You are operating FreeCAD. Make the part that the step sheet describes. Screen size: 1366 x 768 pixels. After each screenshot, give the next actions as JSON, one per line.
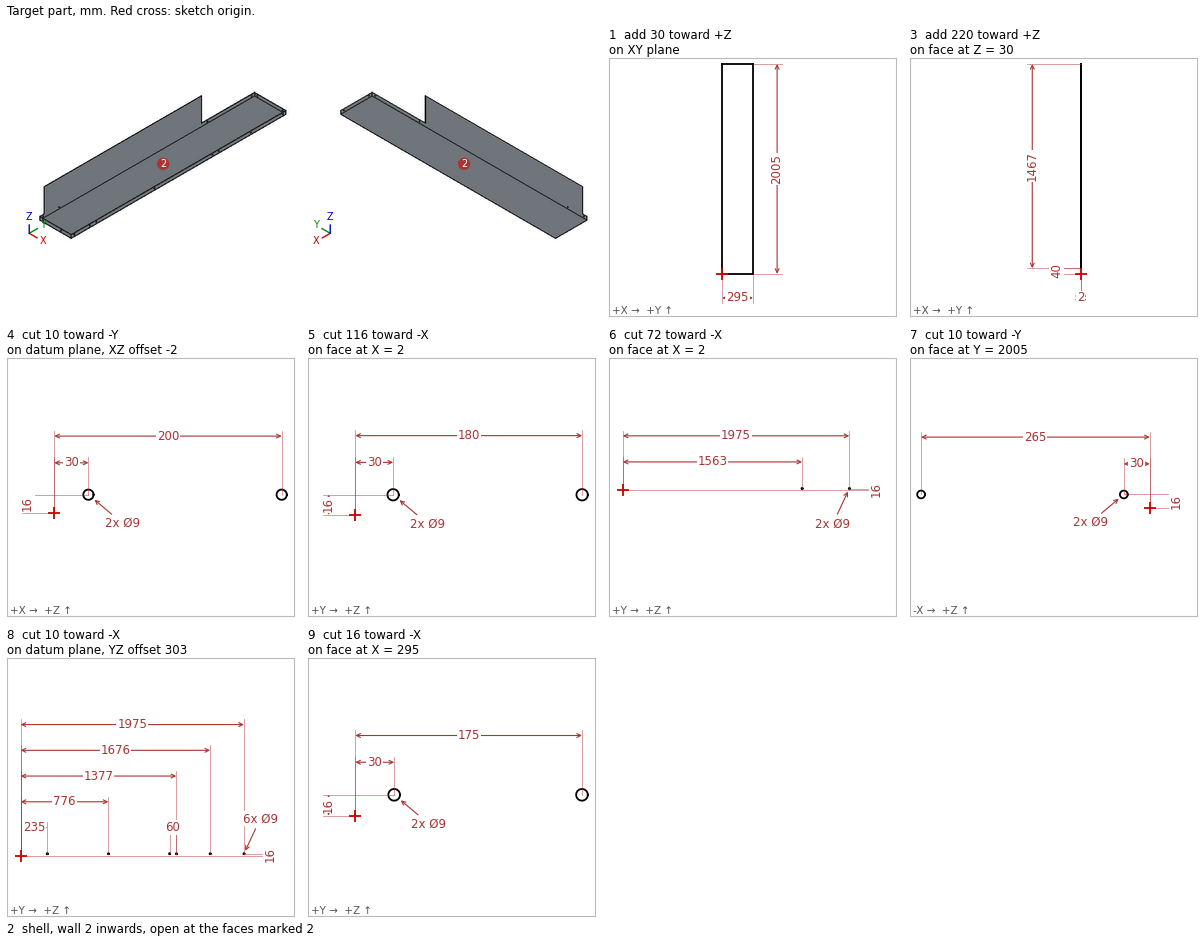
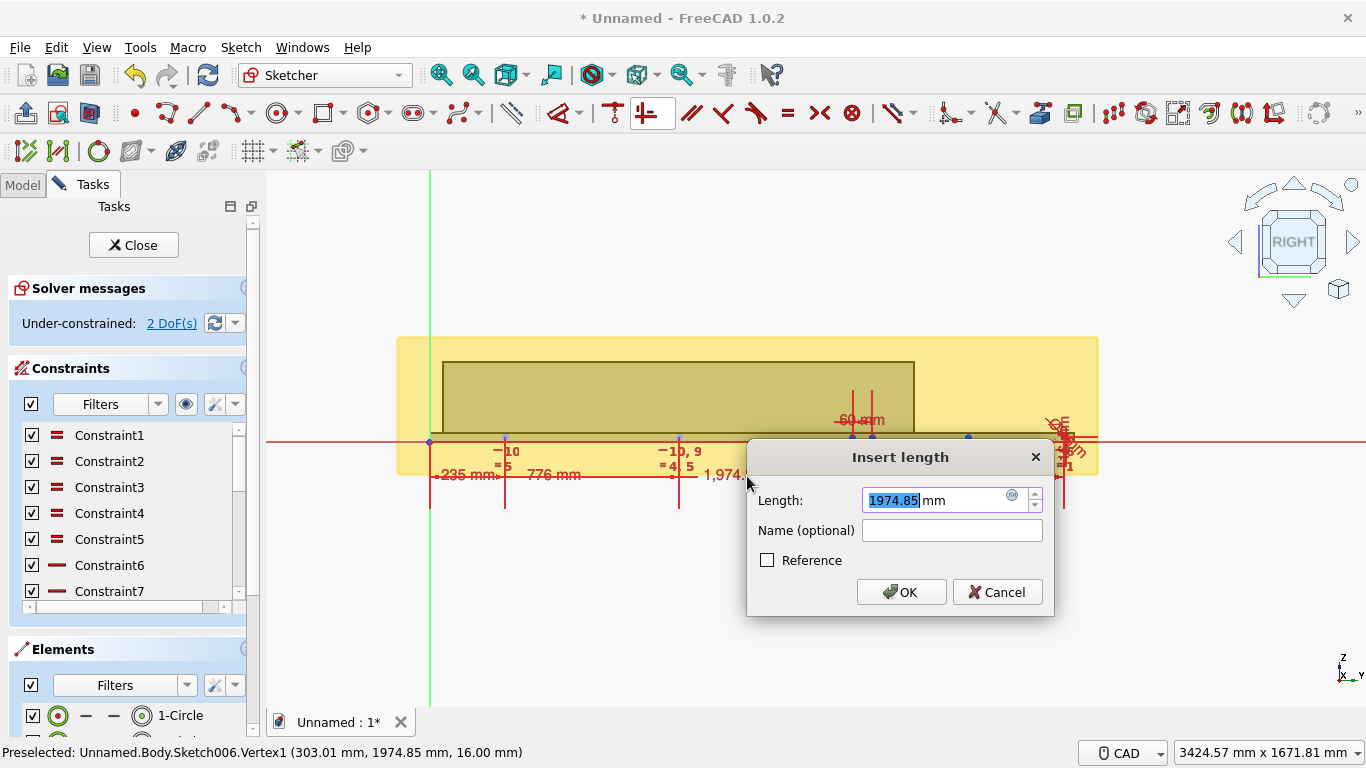
{"action": "type", "text": "1975"}
{"action": "key", "text": "Return"}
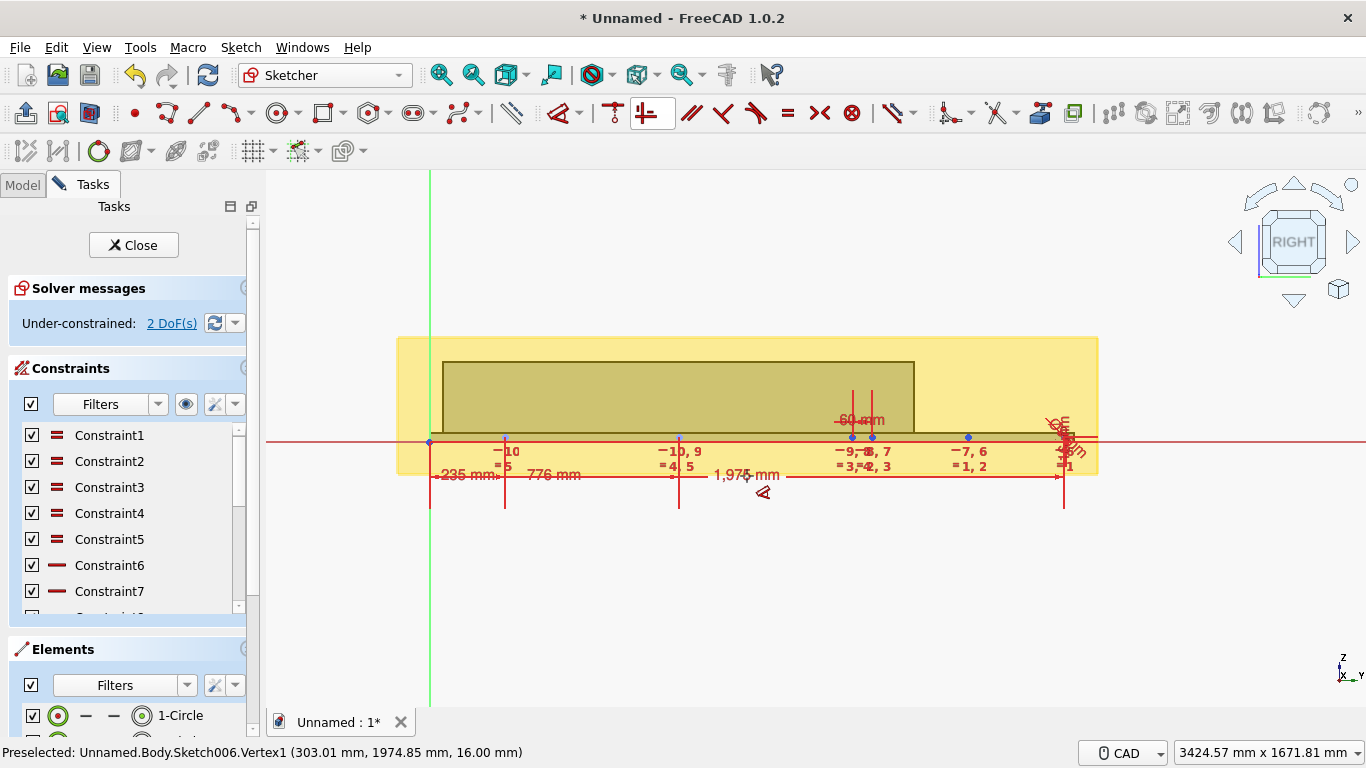
{"action": "left_click", "coordinate": [968, 437]}
{"action": "left_click", "coordinate": [823, 476]}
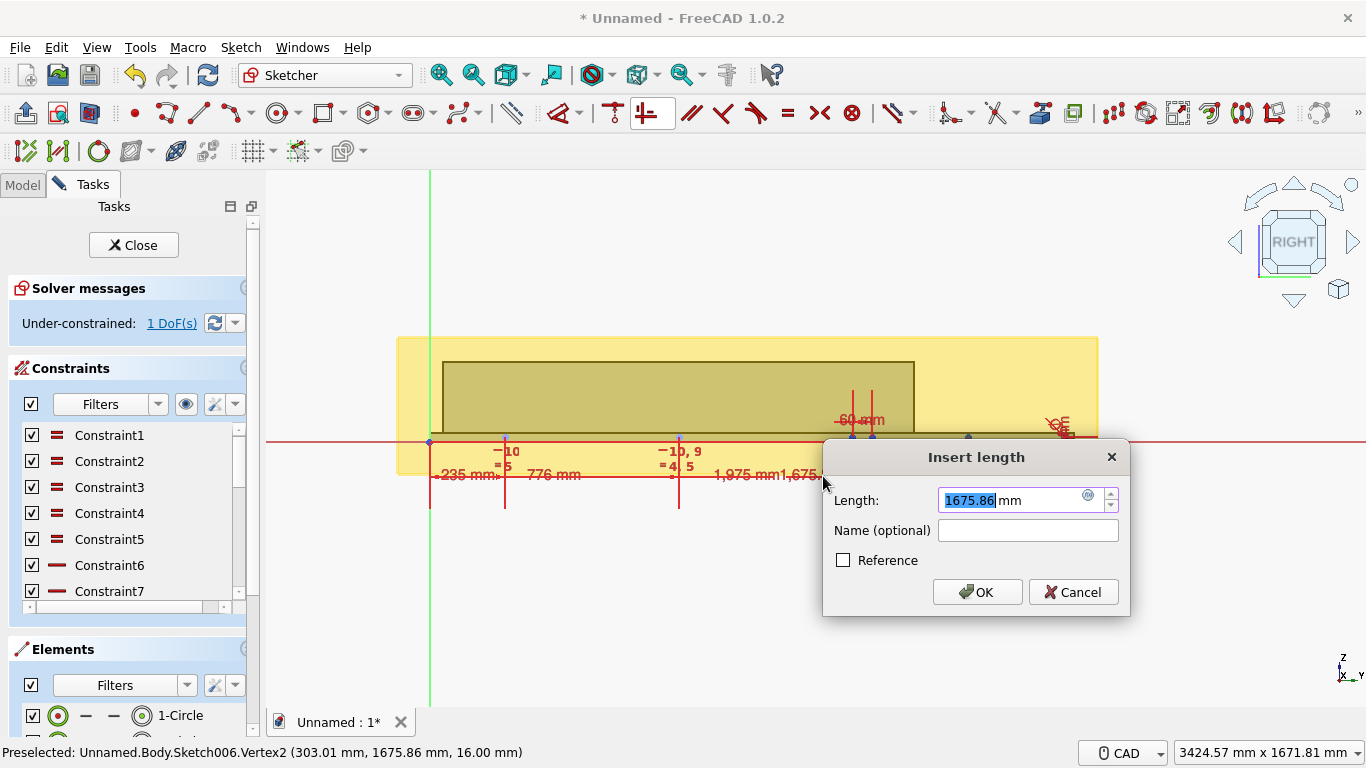
{"action": "type", "text": "1676"}
{"action": "key", "text": "Return"}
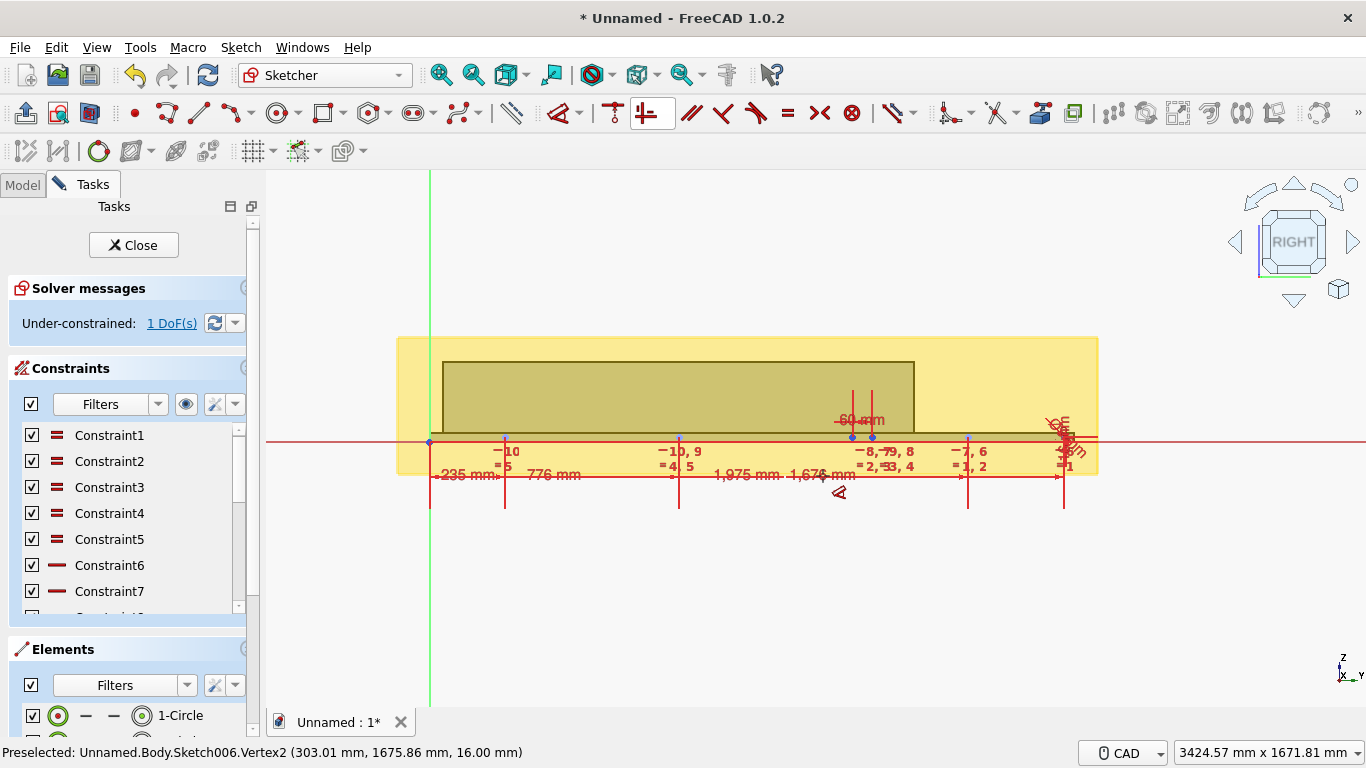
{"action": "left_click", "coordinate": [872, 437]}
{"action": "left_click", "coordinate": [651, 476]}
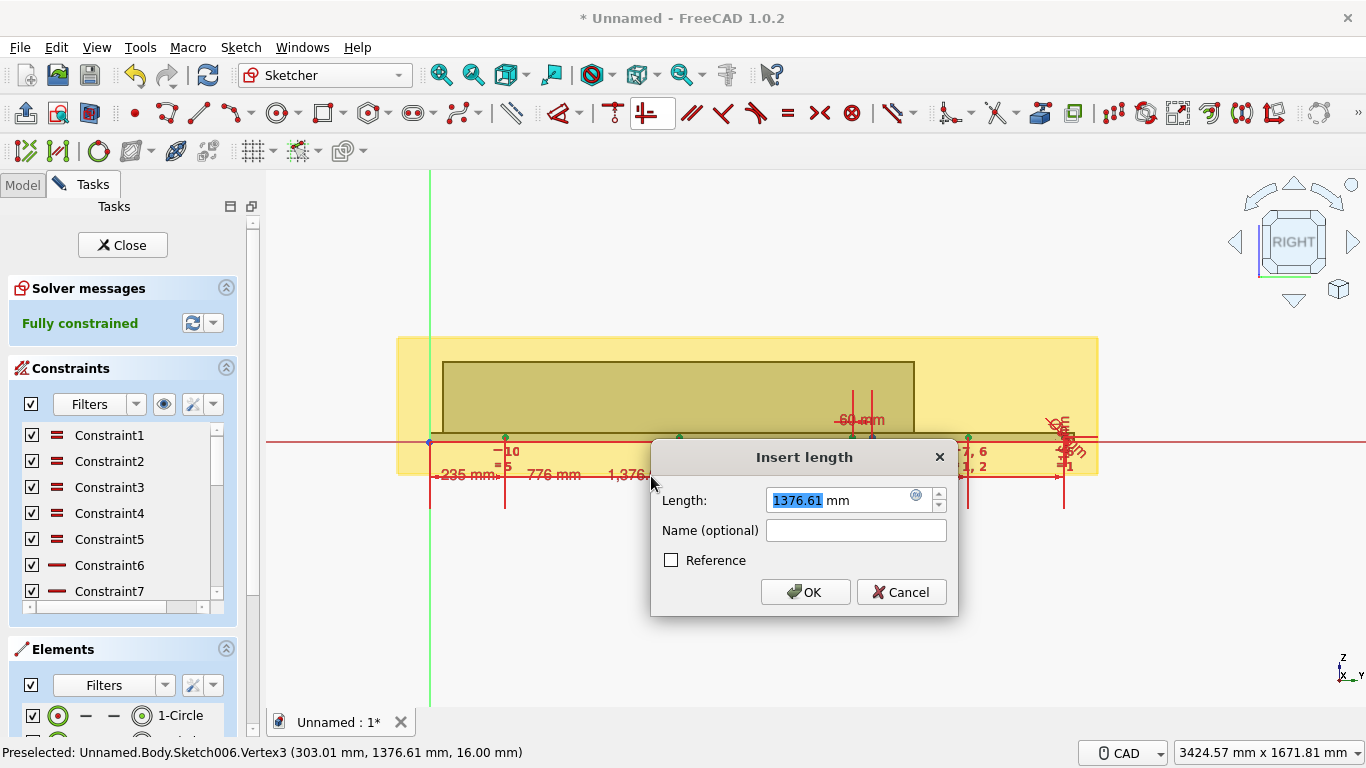
{"action": "type", "text": "1377"}
{"action": "key", "text": "Return"}
{"action": "key", "text": "Escape"}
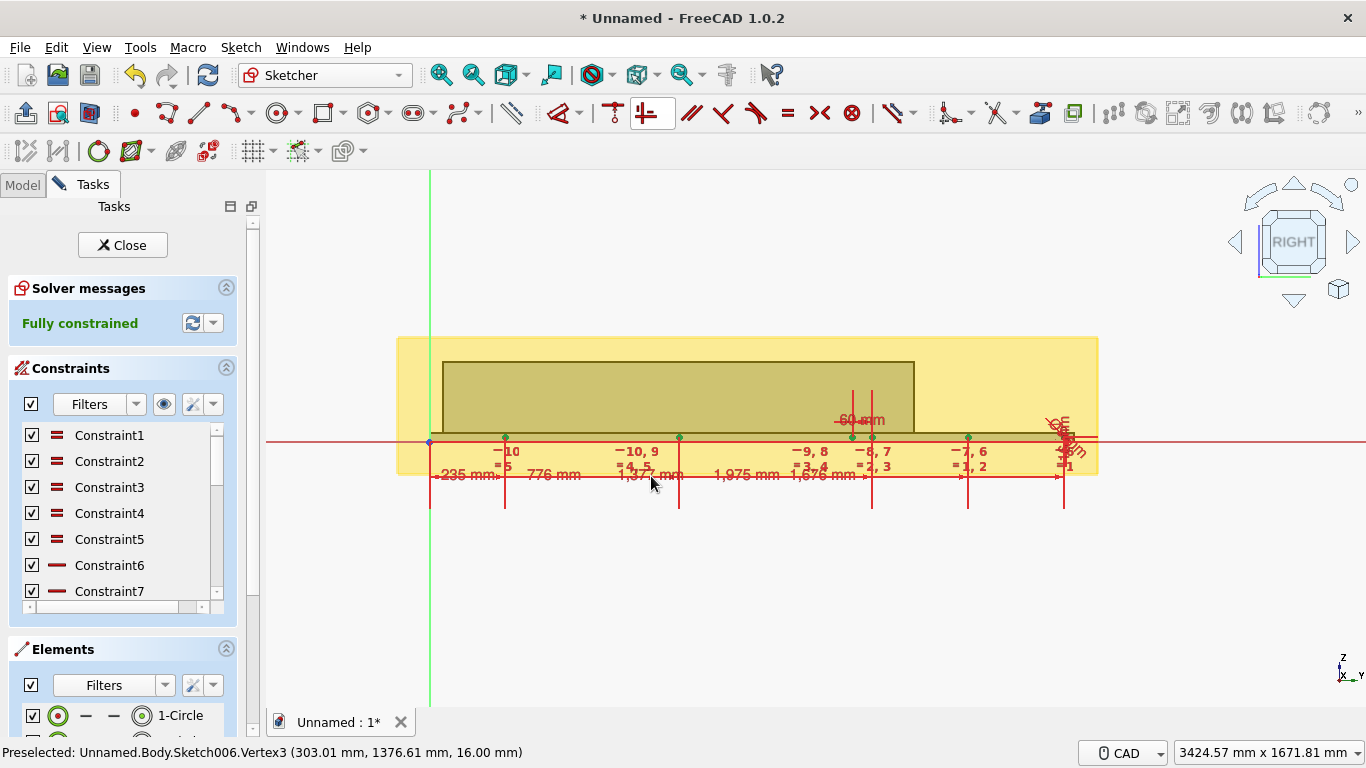
{"action": "left_click", "coordinate": [123, 245]}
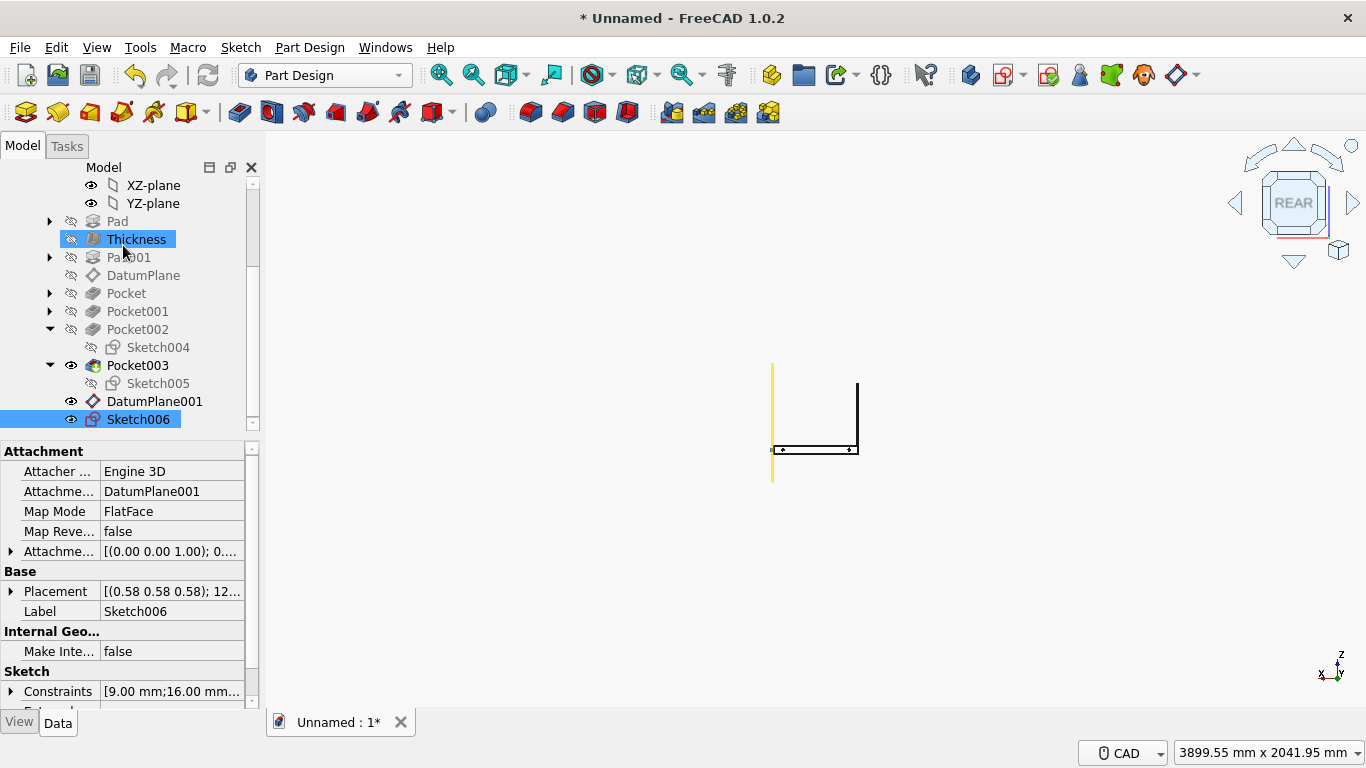
{"action": "left_click", "coordinate": [240, 112]}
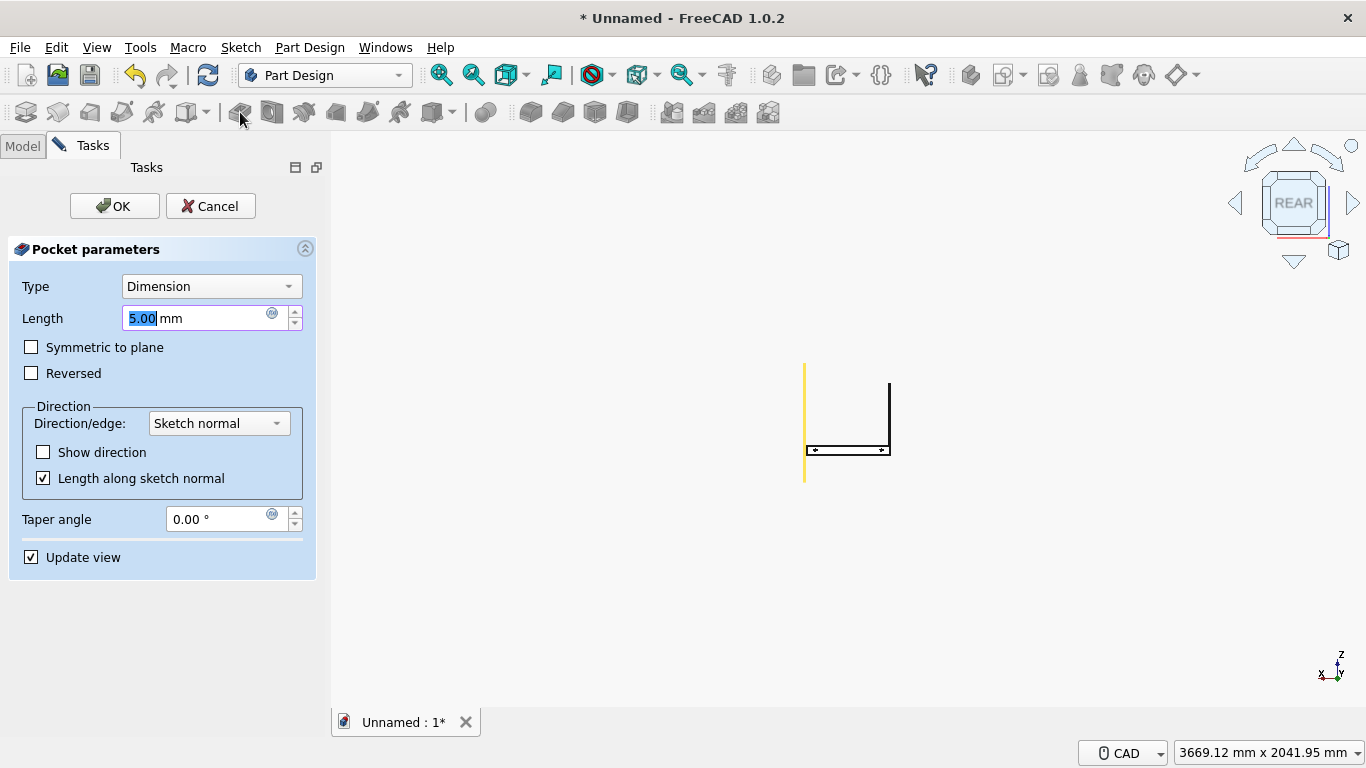
{"action": "type", "text": "10"}
{"action": "key", "text": "Tab"}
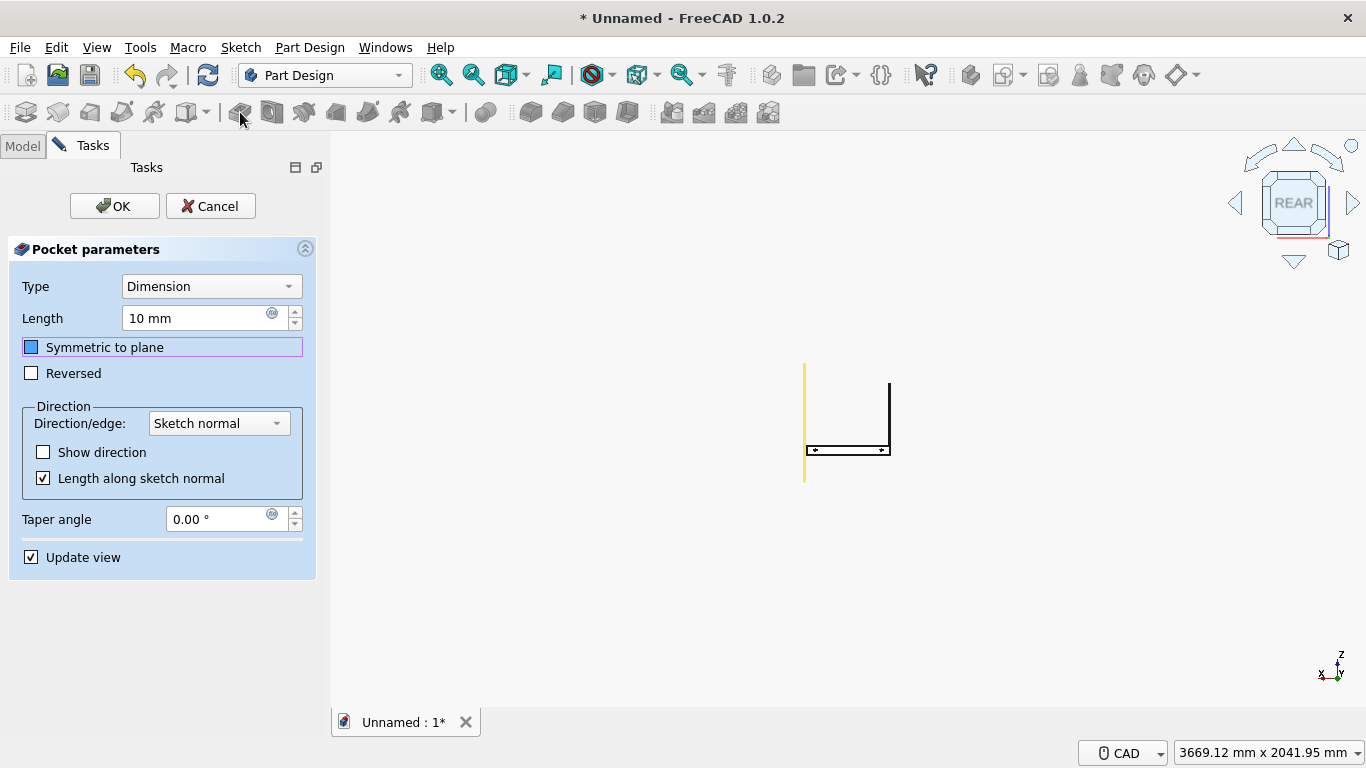
{"action": "left_click", "coordinate": [115, 206]}